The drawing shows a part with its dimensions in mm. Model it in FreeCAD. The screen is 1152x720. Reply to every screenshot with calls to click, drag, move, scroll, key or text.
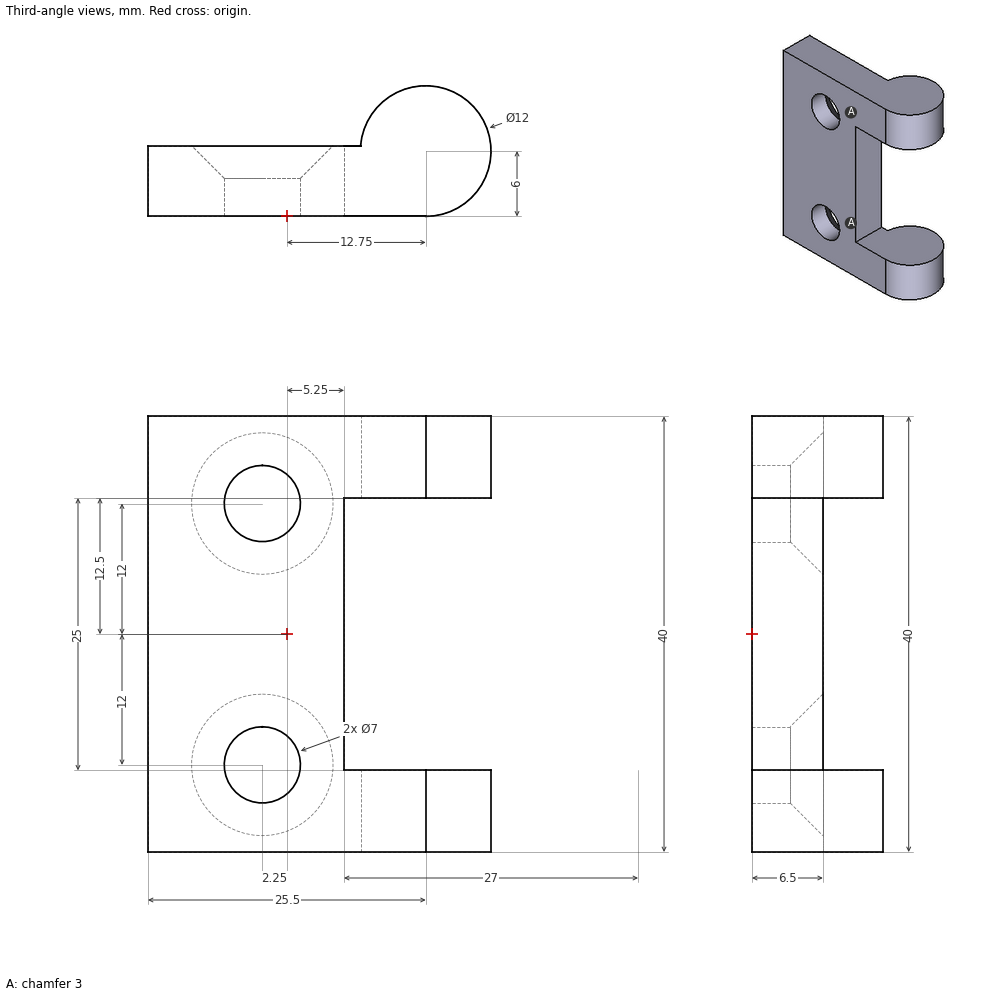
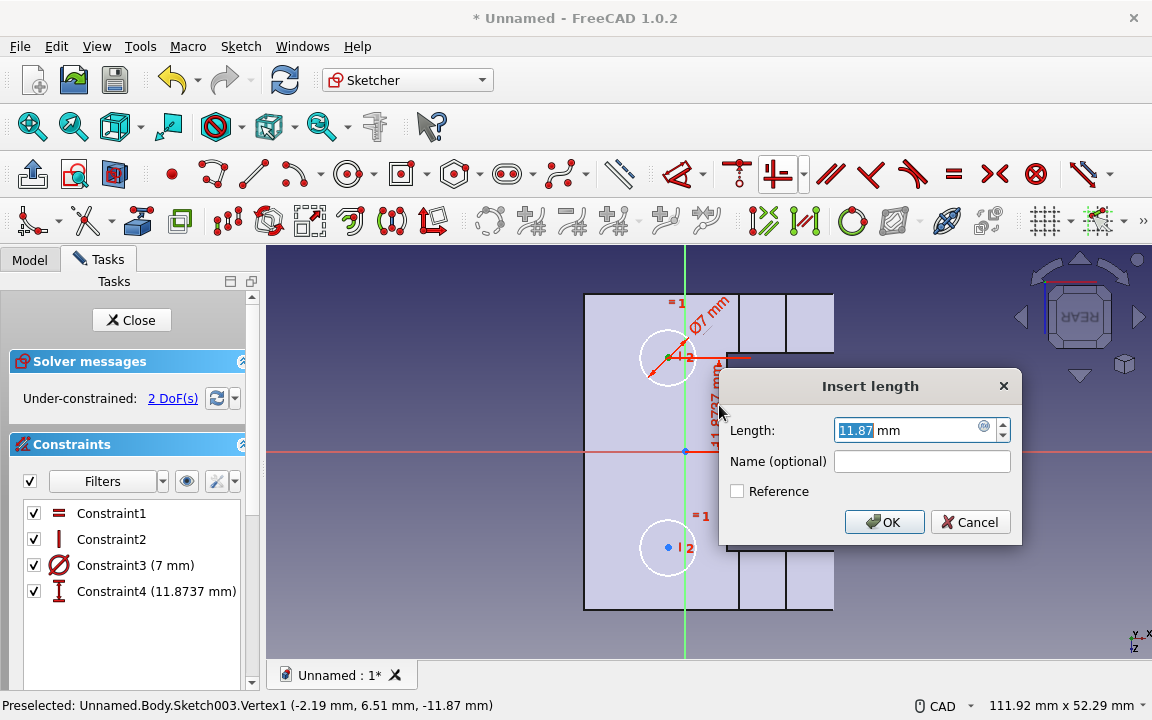
text(12)
key(Return)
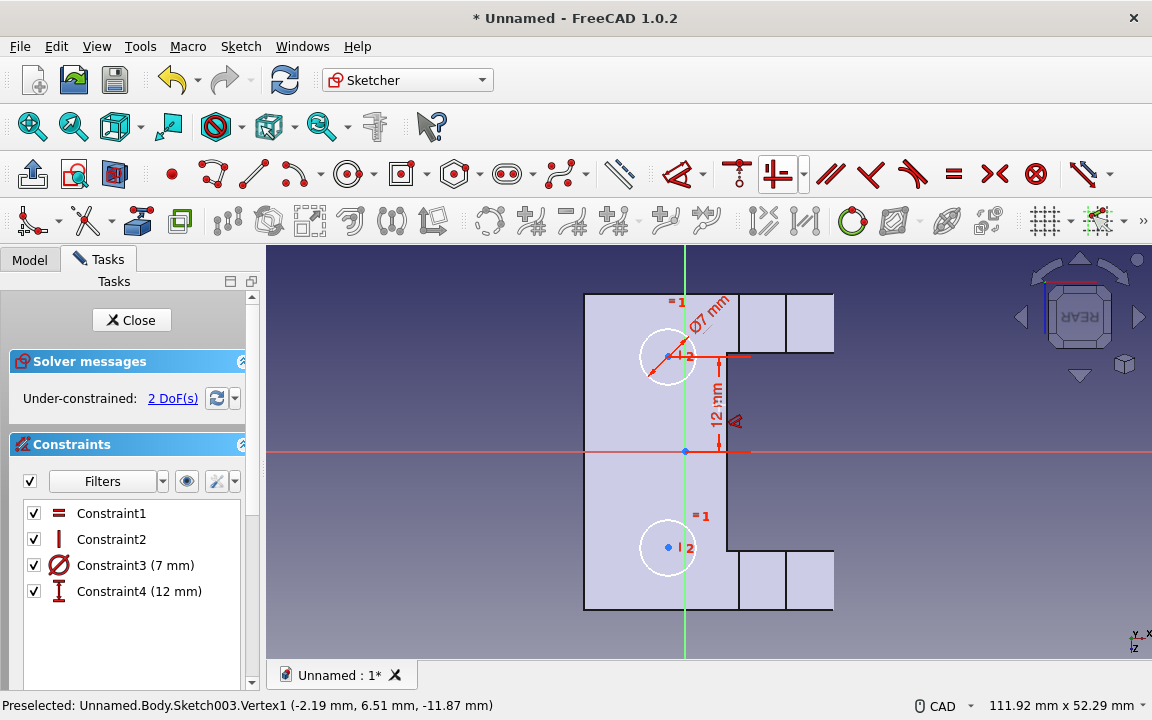
click(668, 548)
click(719, 500)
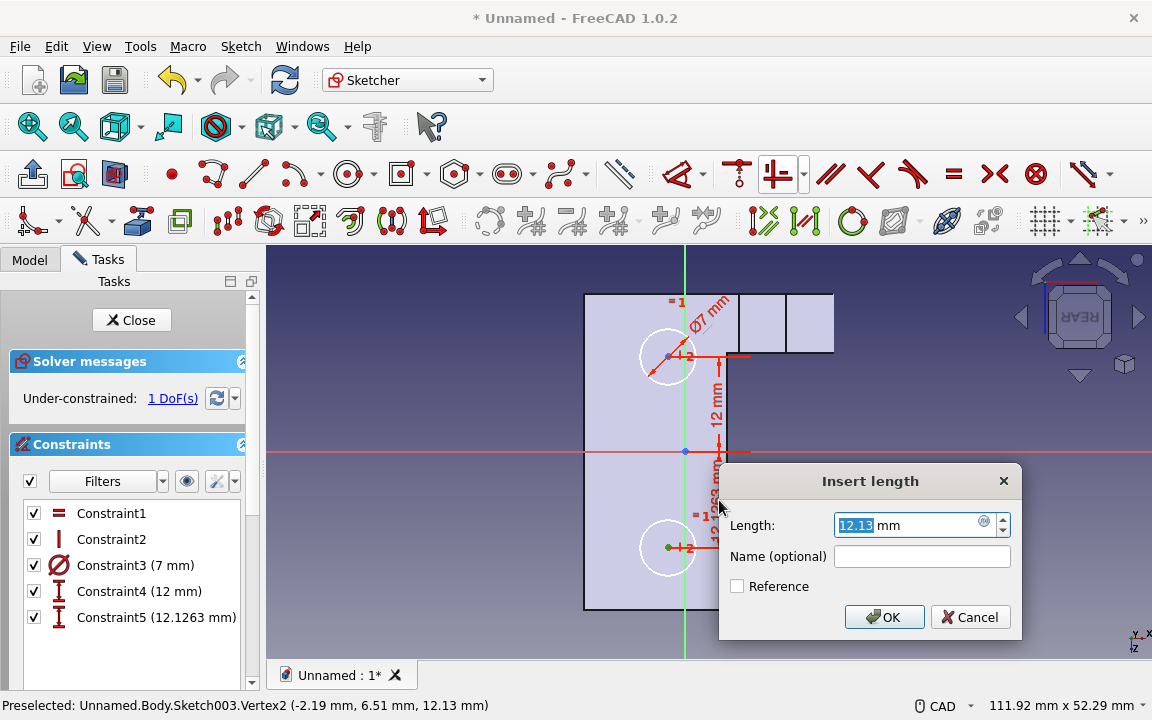
text(12)
key(Return)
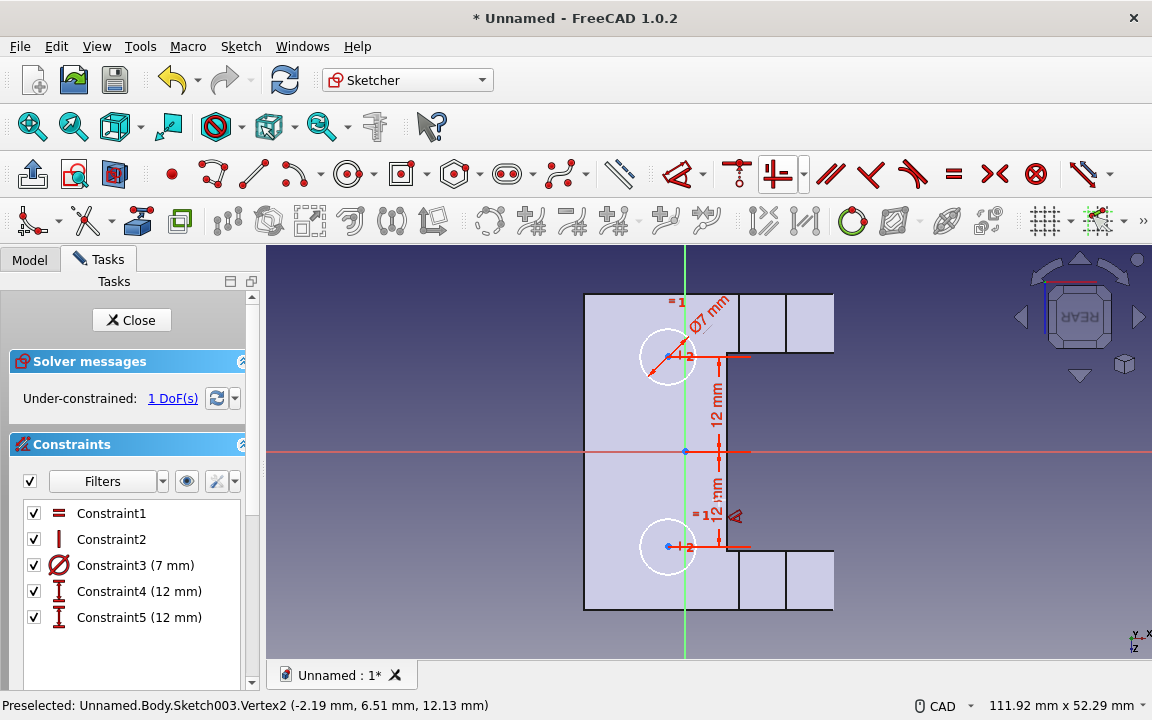
scroll(668, 357, up, 5)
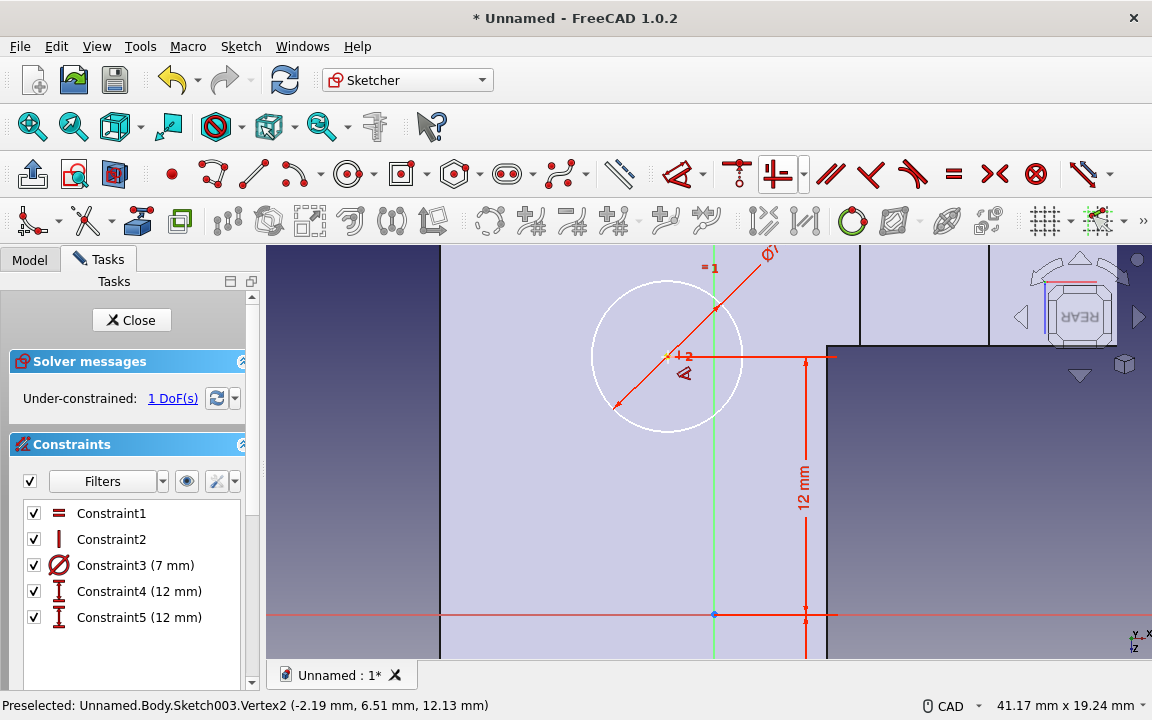
click(667, 357)
click(691, 323)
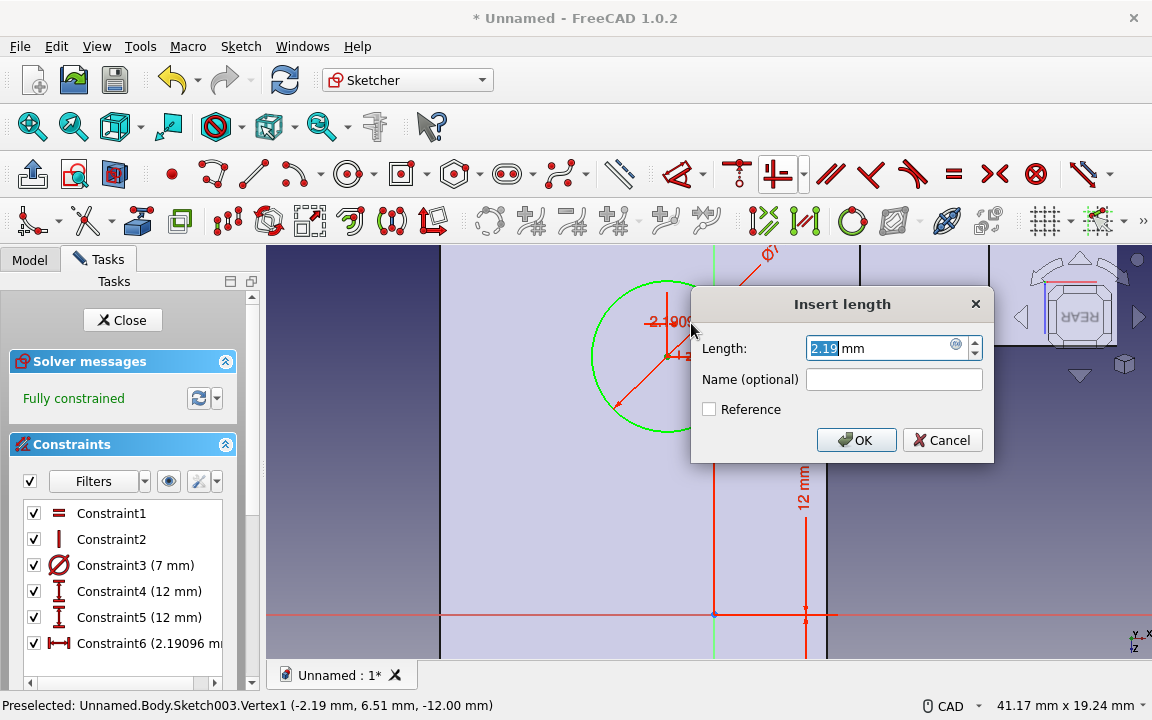
text(2.25)
key(Return)
key(Escape)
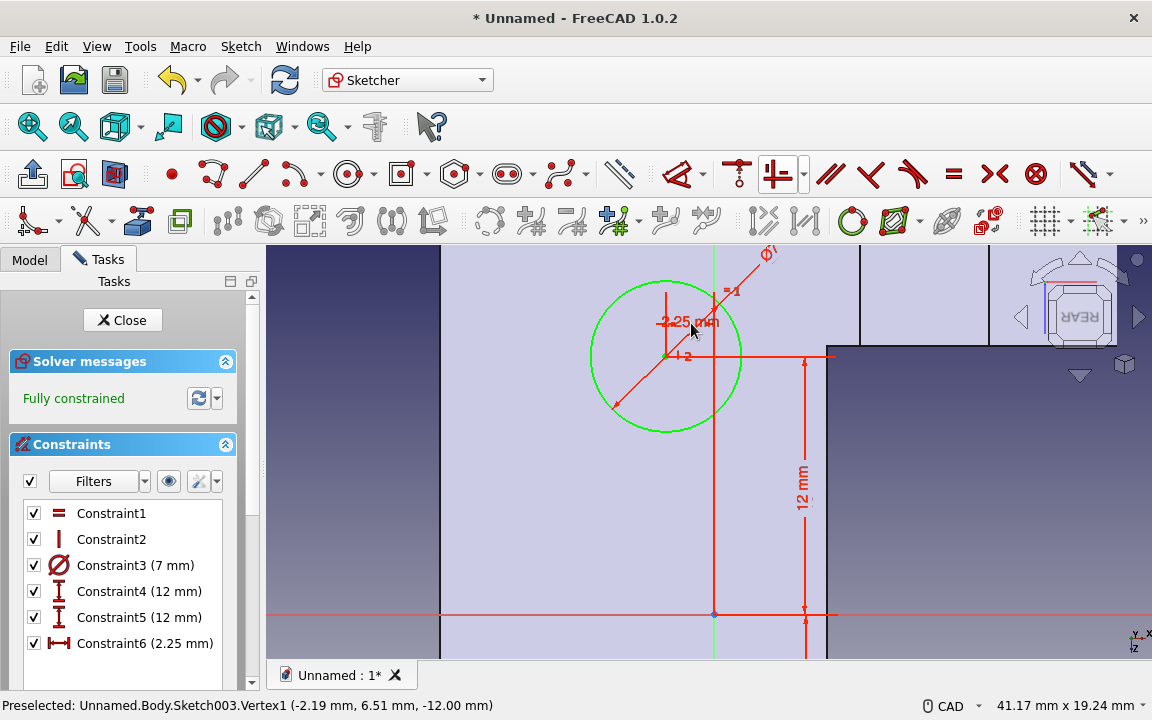
click(123, 320)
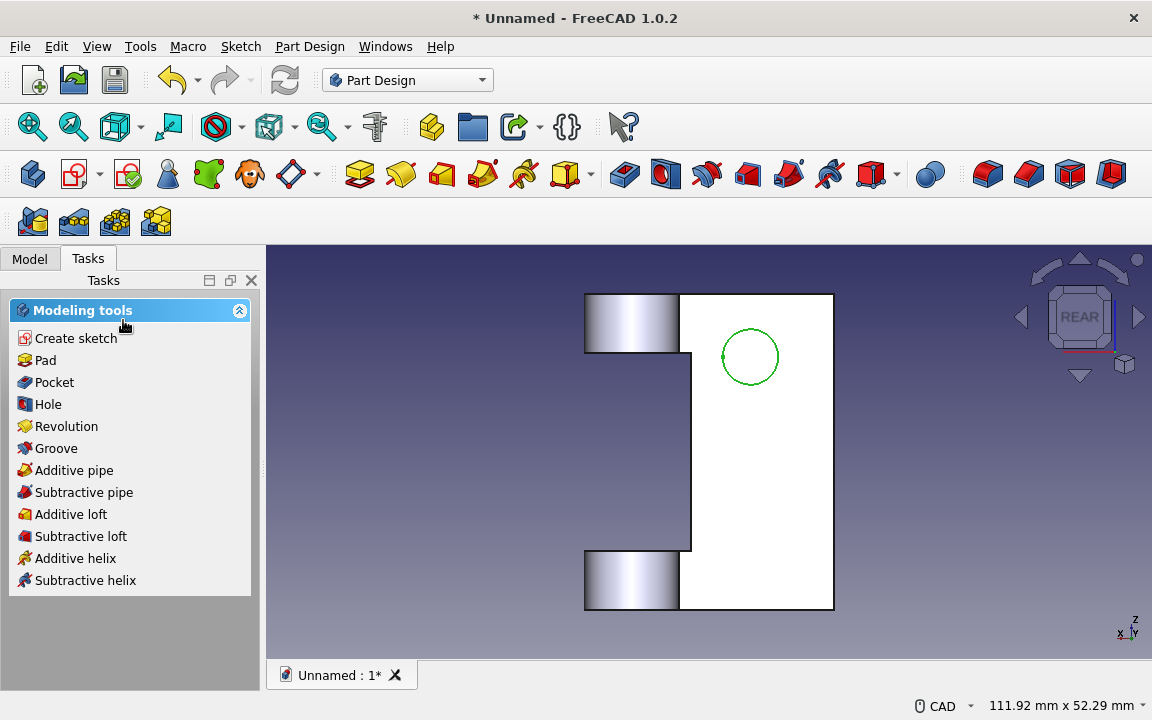
click(625, 174)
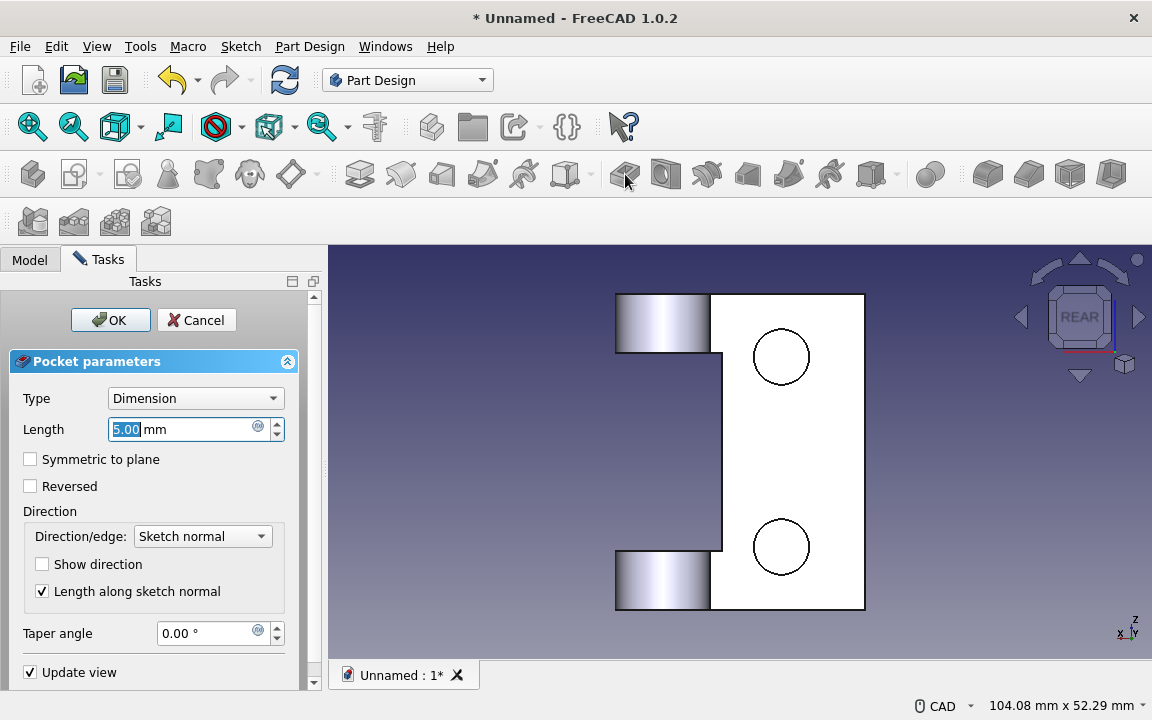
click(196, 398)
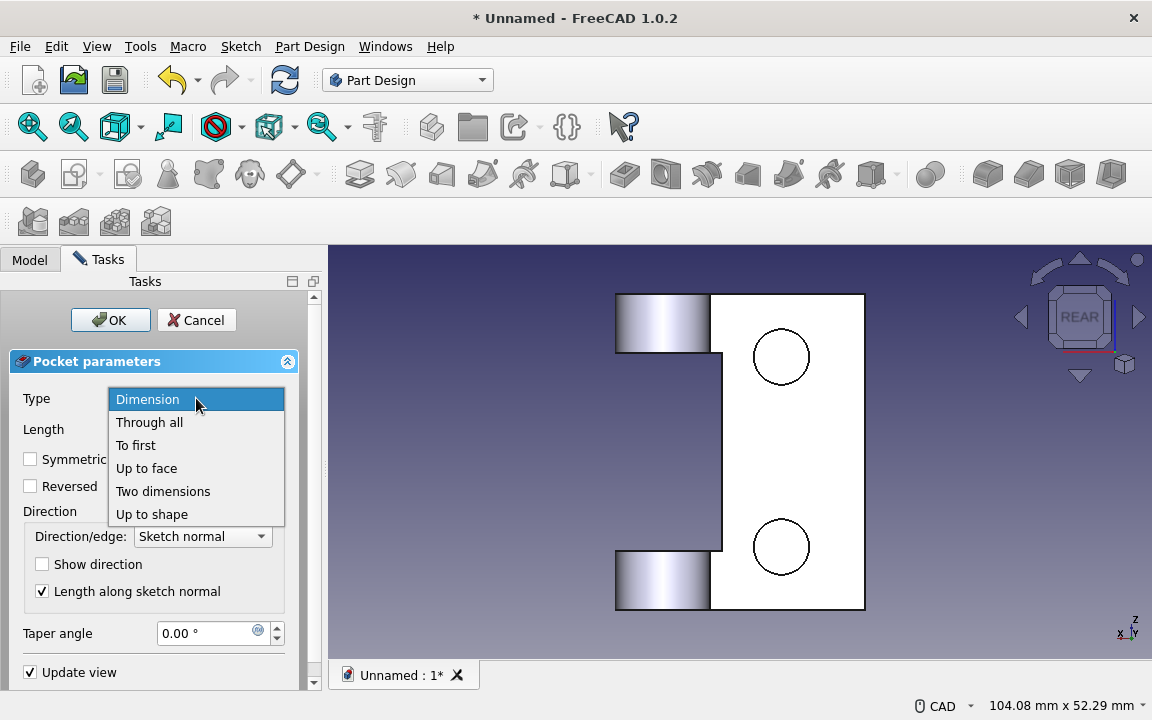
click(194, 422)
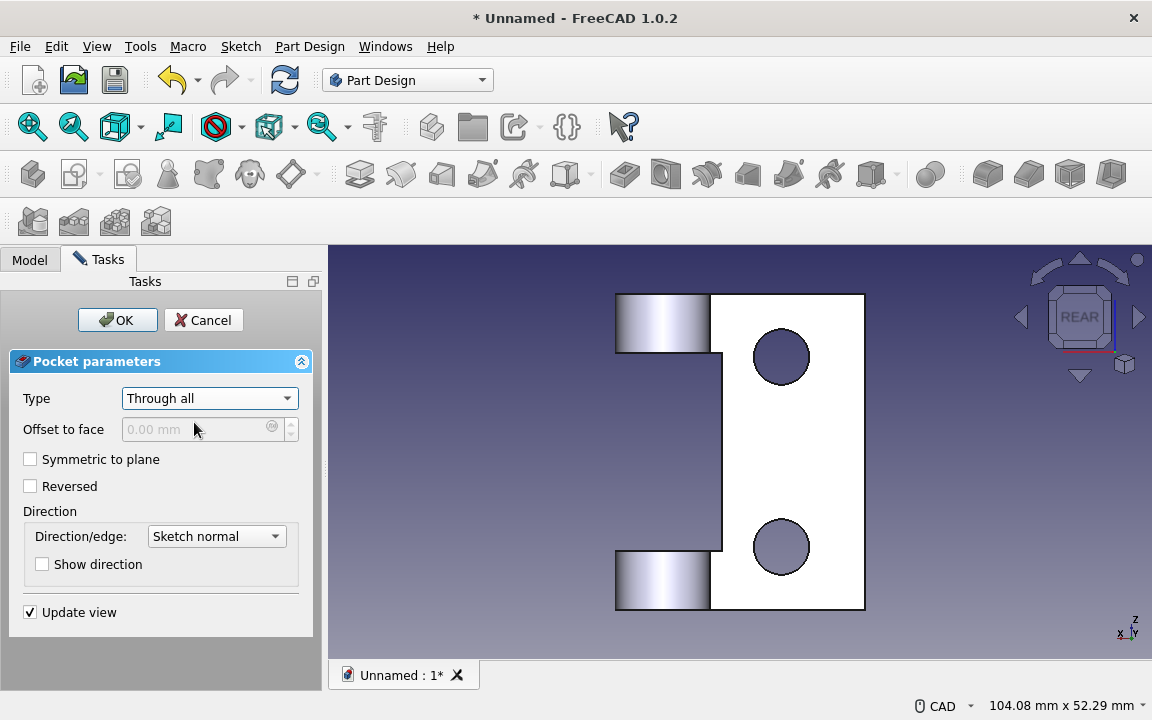
click(118, 320)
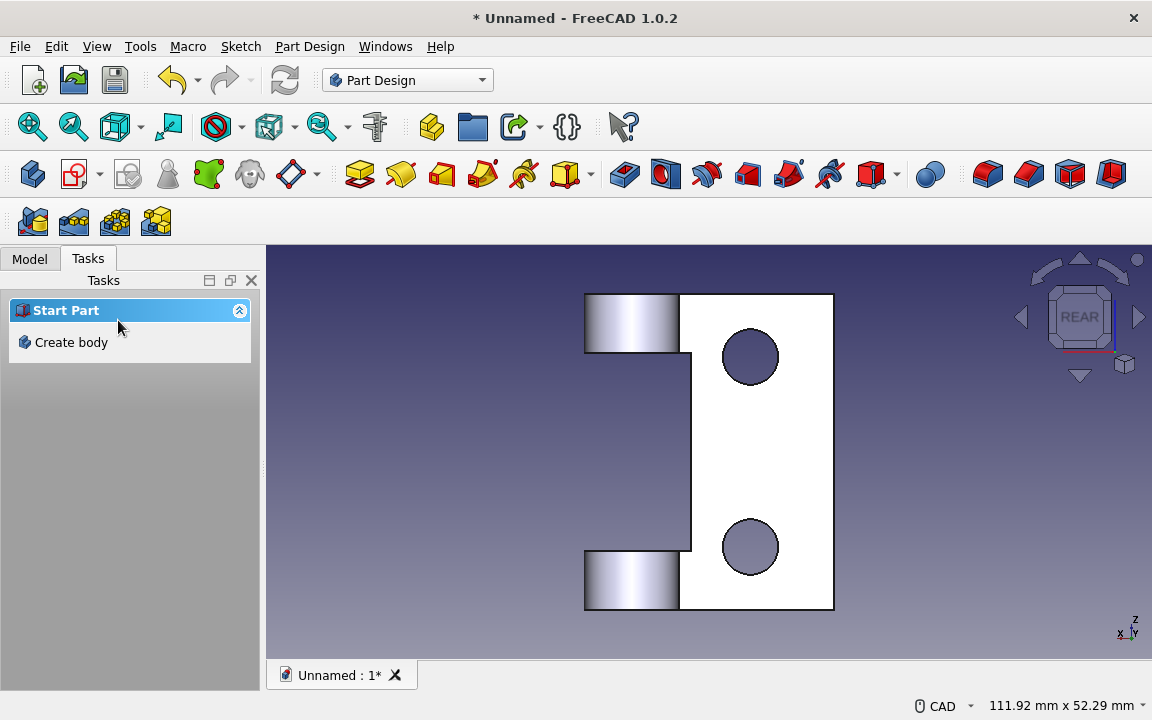
click(773, 530)